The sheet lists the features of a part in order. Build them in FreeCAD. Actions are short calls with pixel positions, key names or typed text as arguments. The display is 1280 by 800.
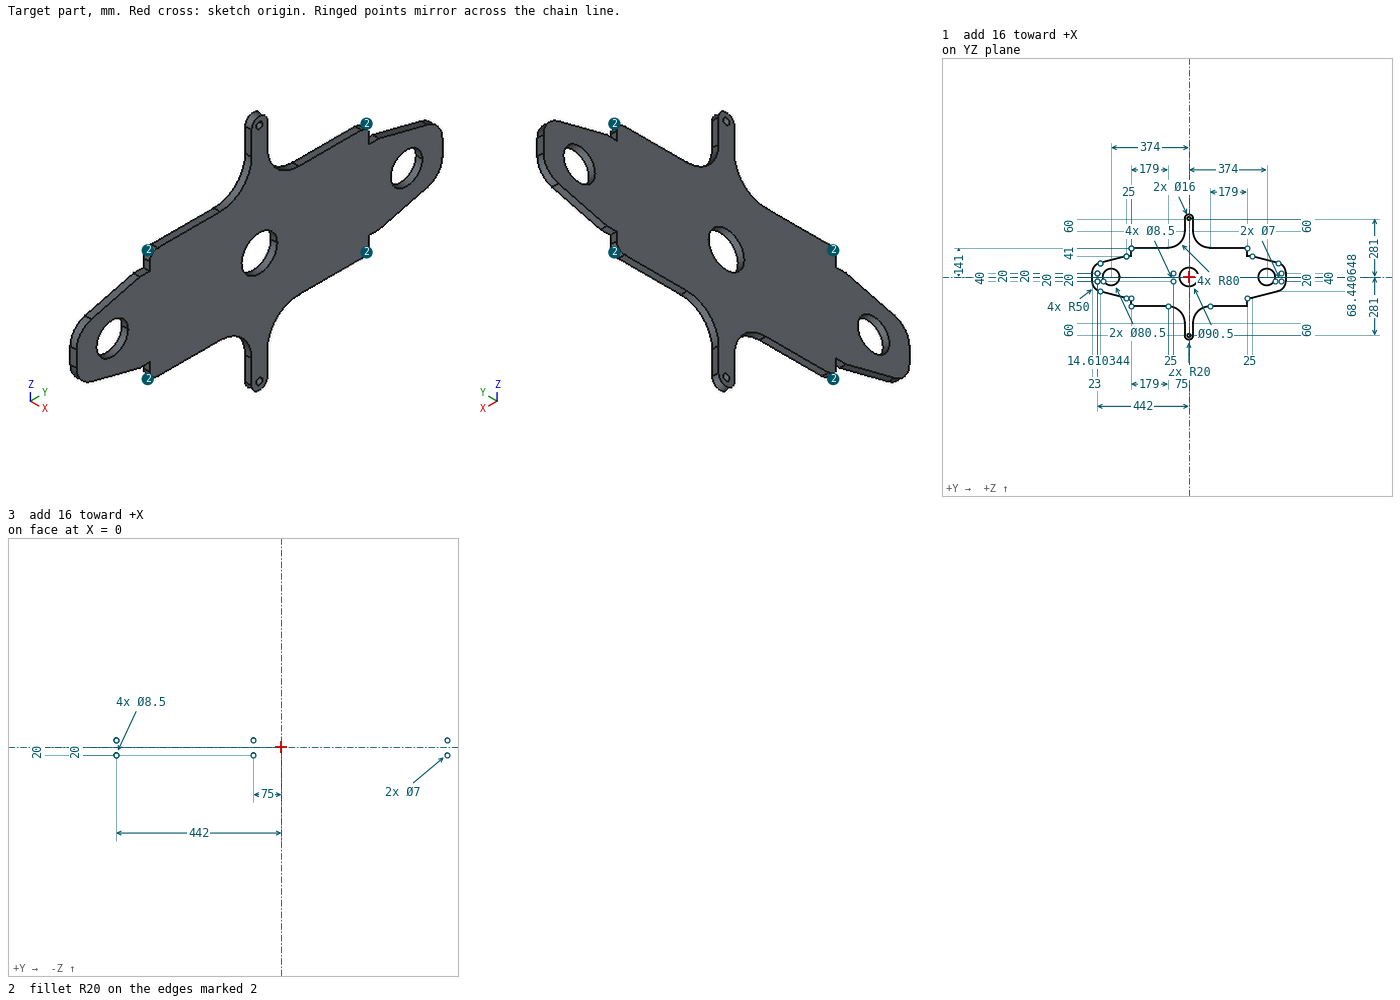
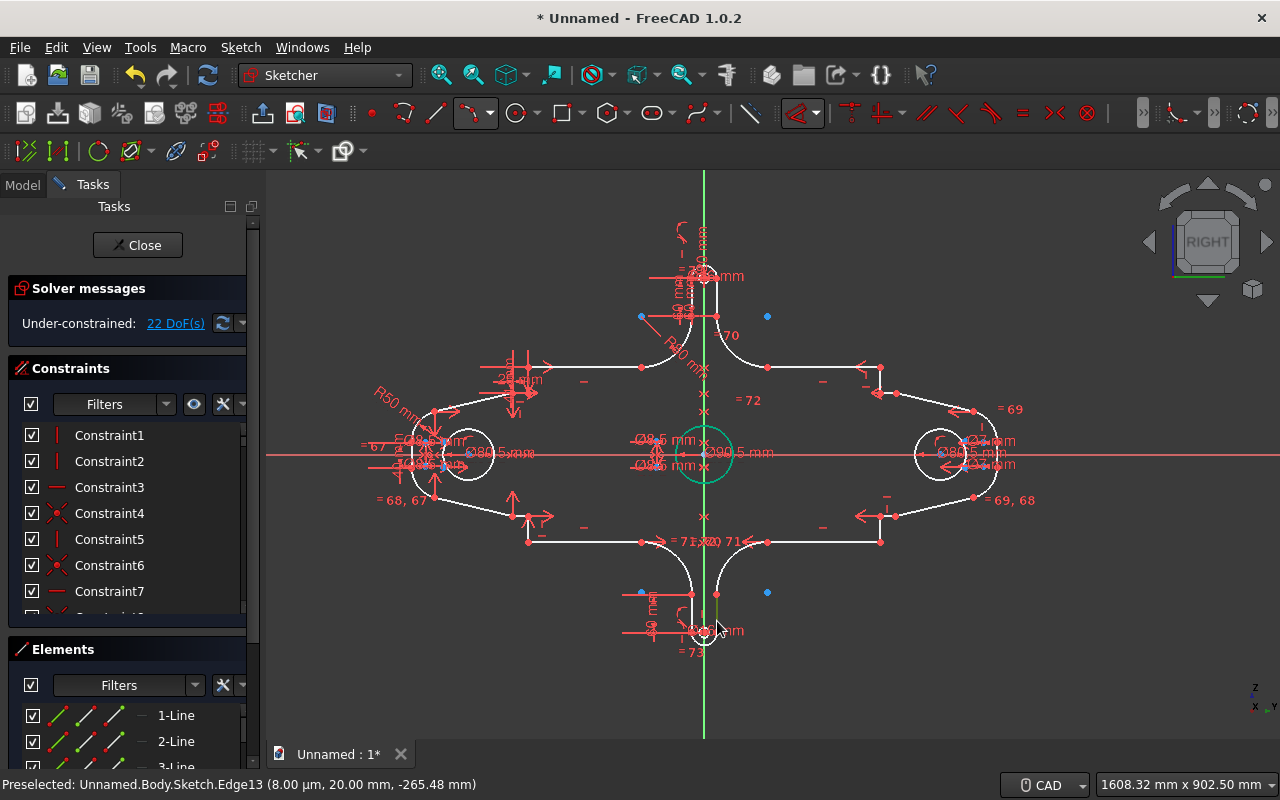
key(i)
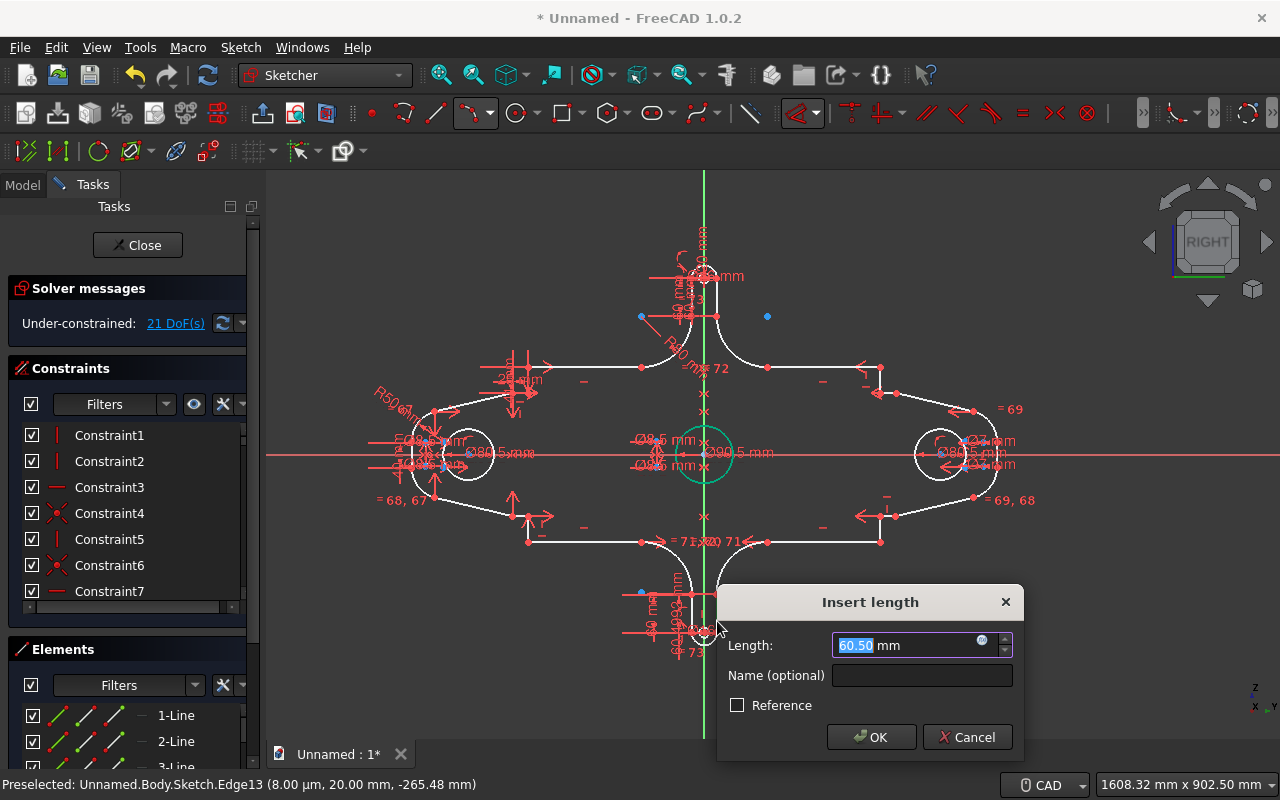
text(60)
key(Return)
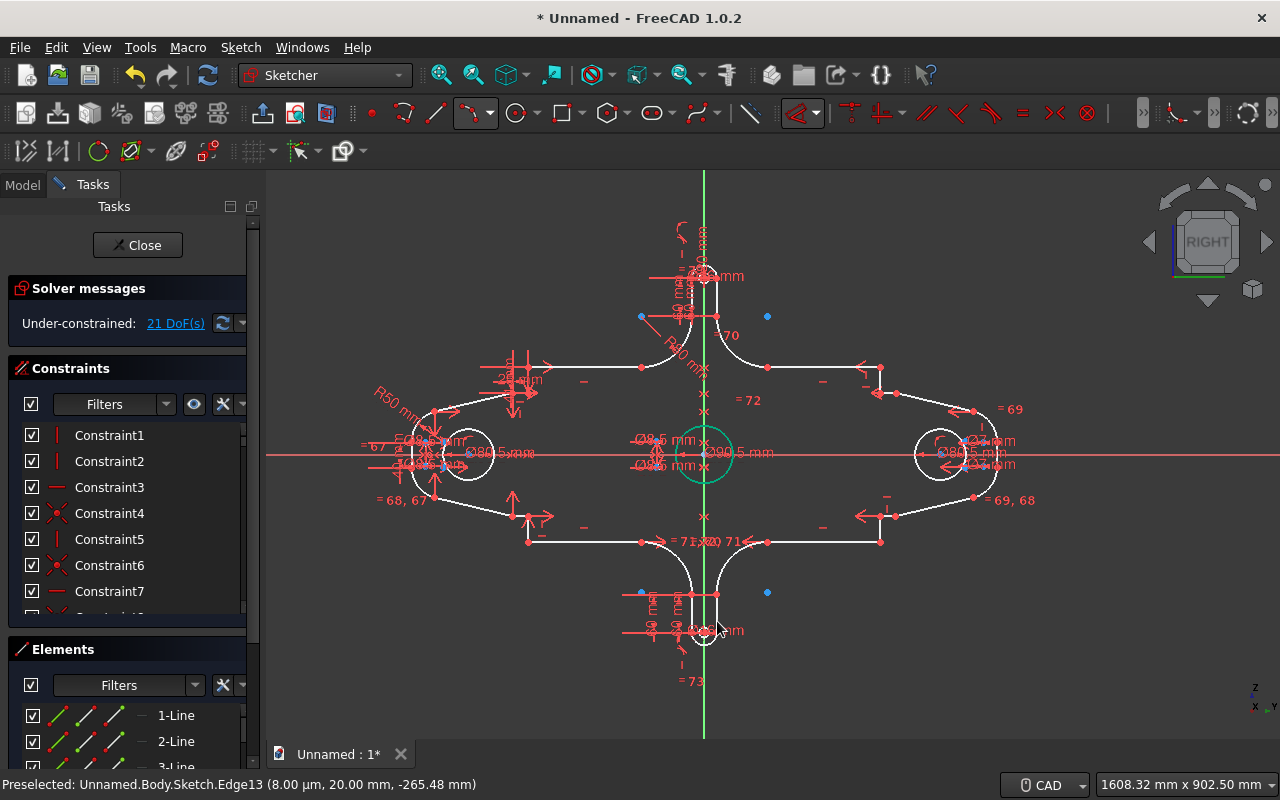
scroll(888, 516, up, 5)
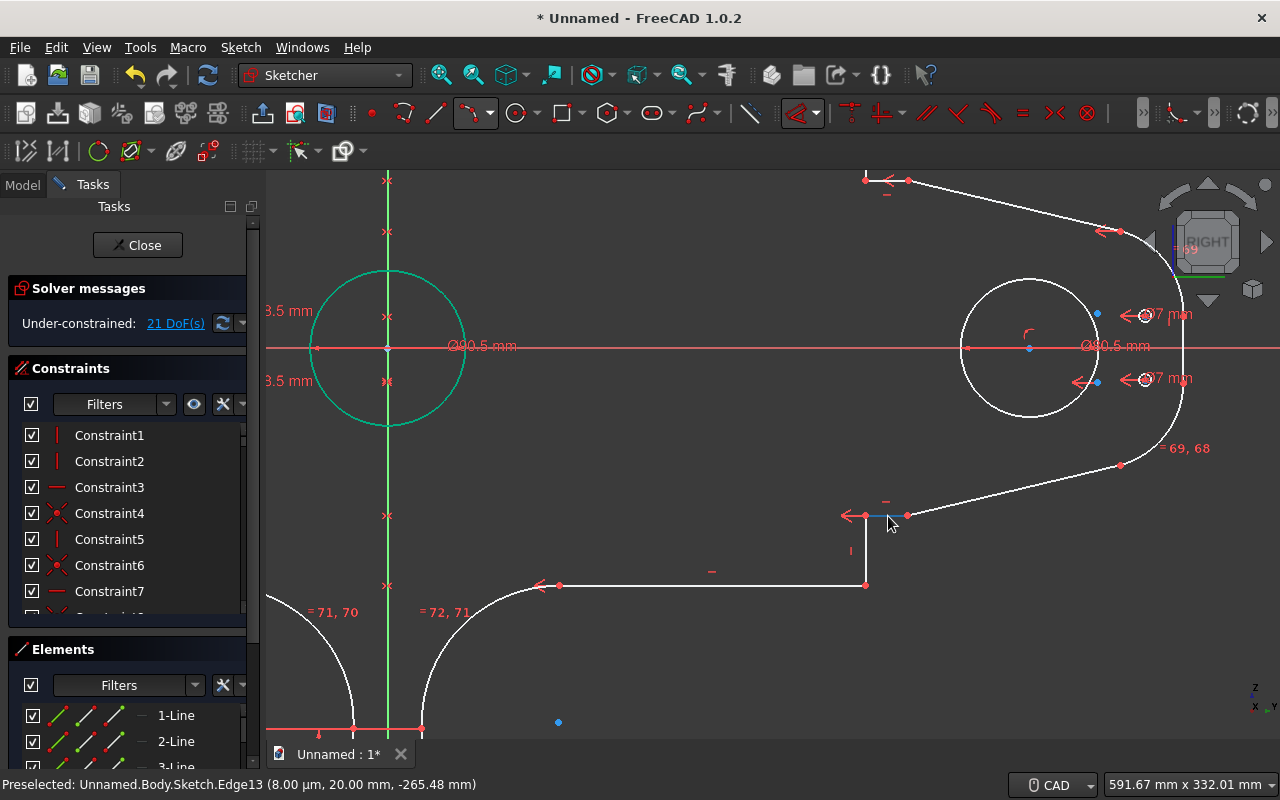
click(887, 516)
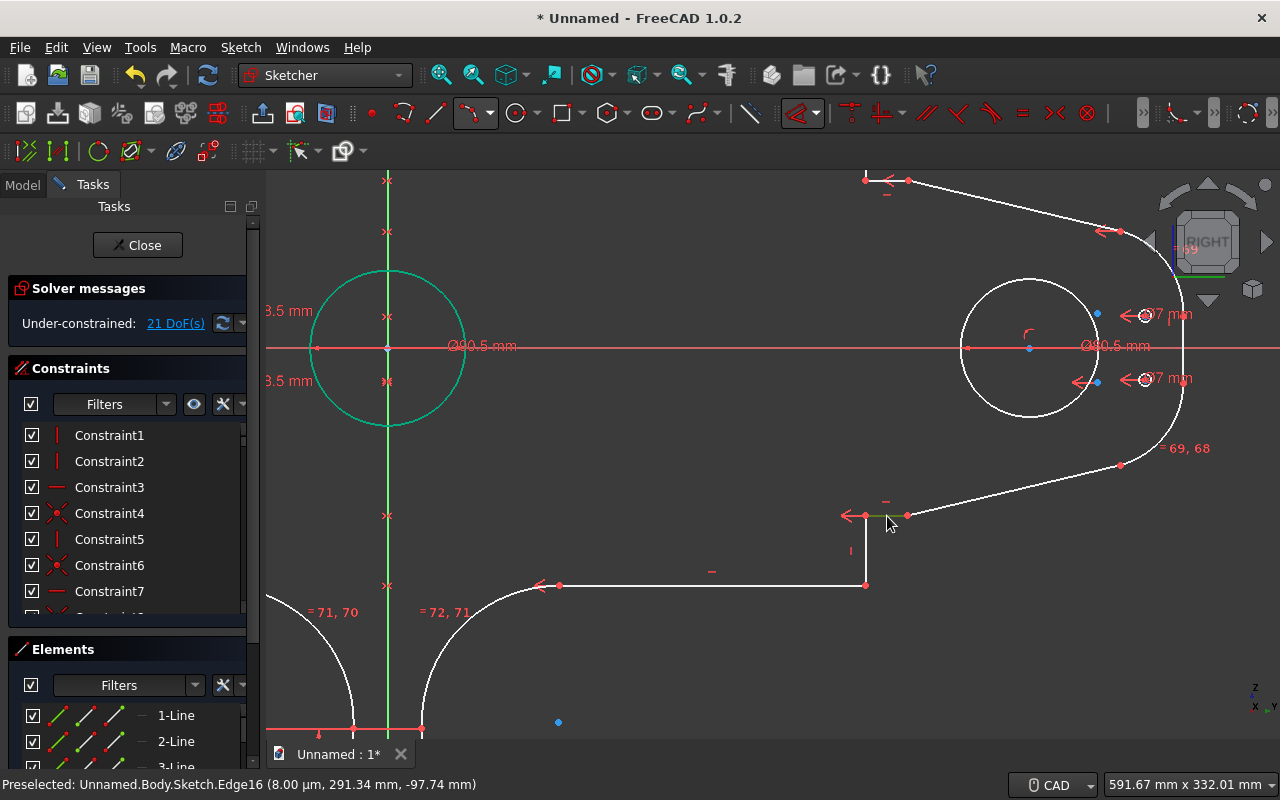
key(l)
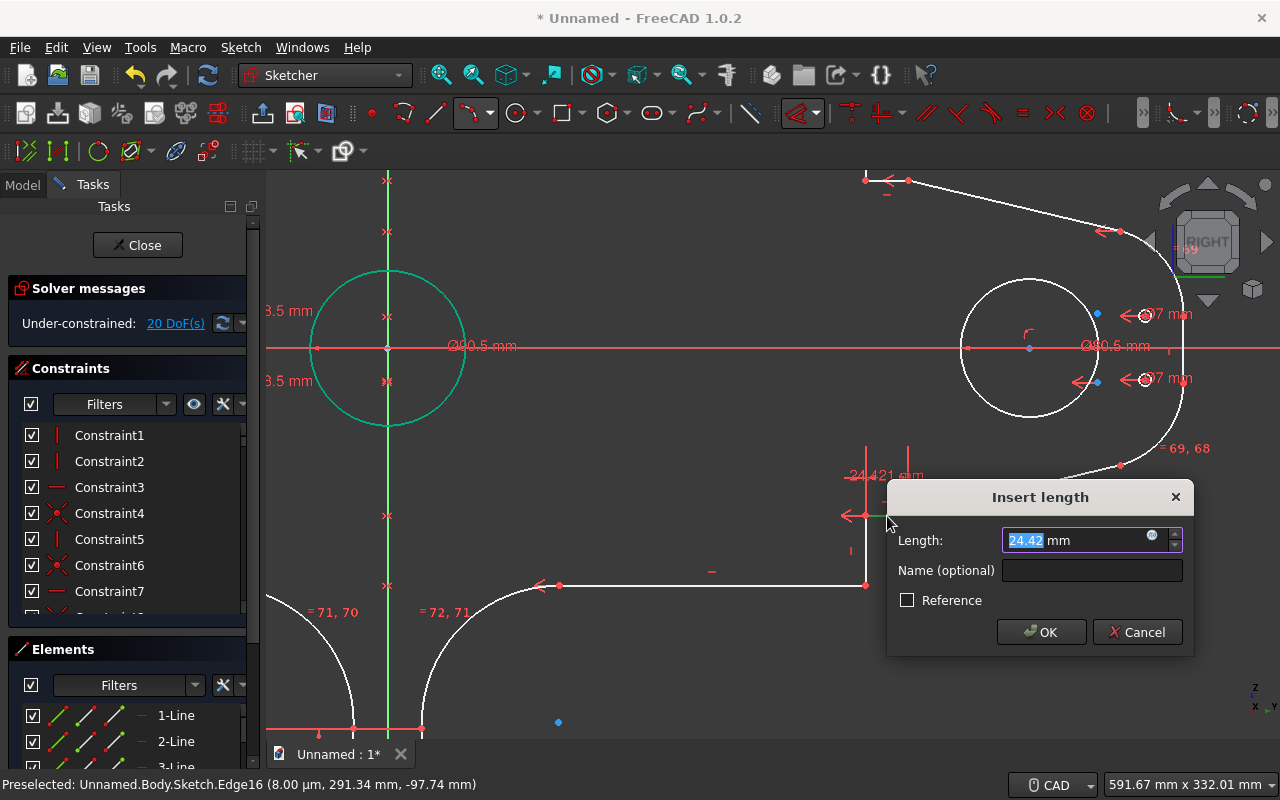
text(25)
key(Return)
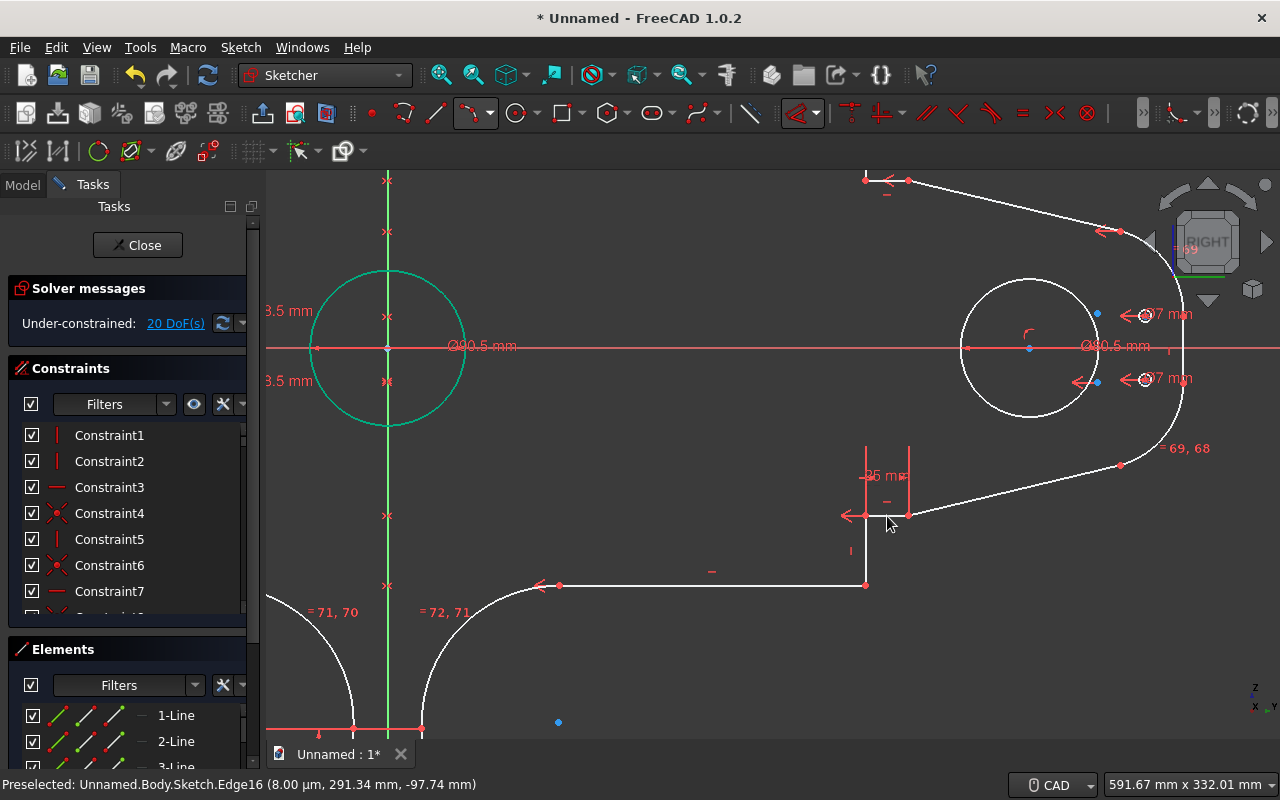
scroll(889, 516, down, 5)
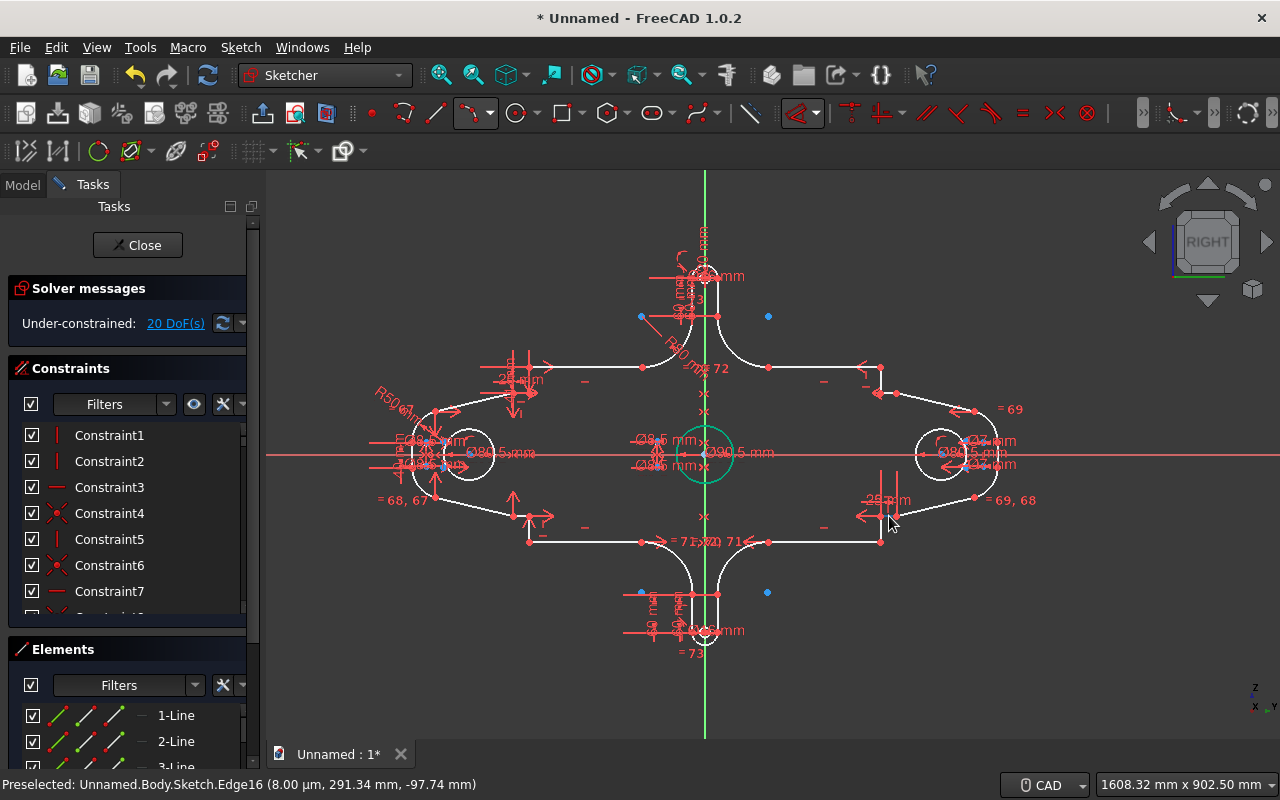
scroll(998, 460, up, 5)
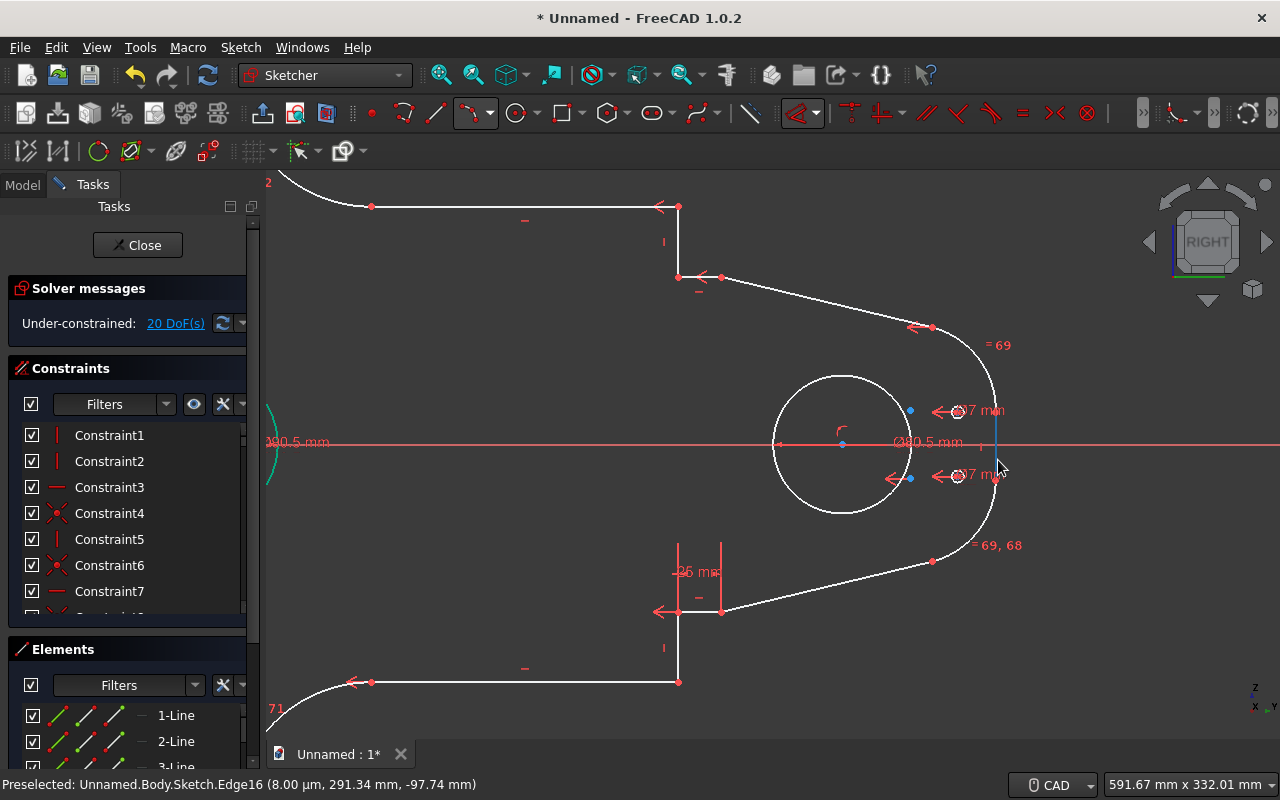
click(996, 460)